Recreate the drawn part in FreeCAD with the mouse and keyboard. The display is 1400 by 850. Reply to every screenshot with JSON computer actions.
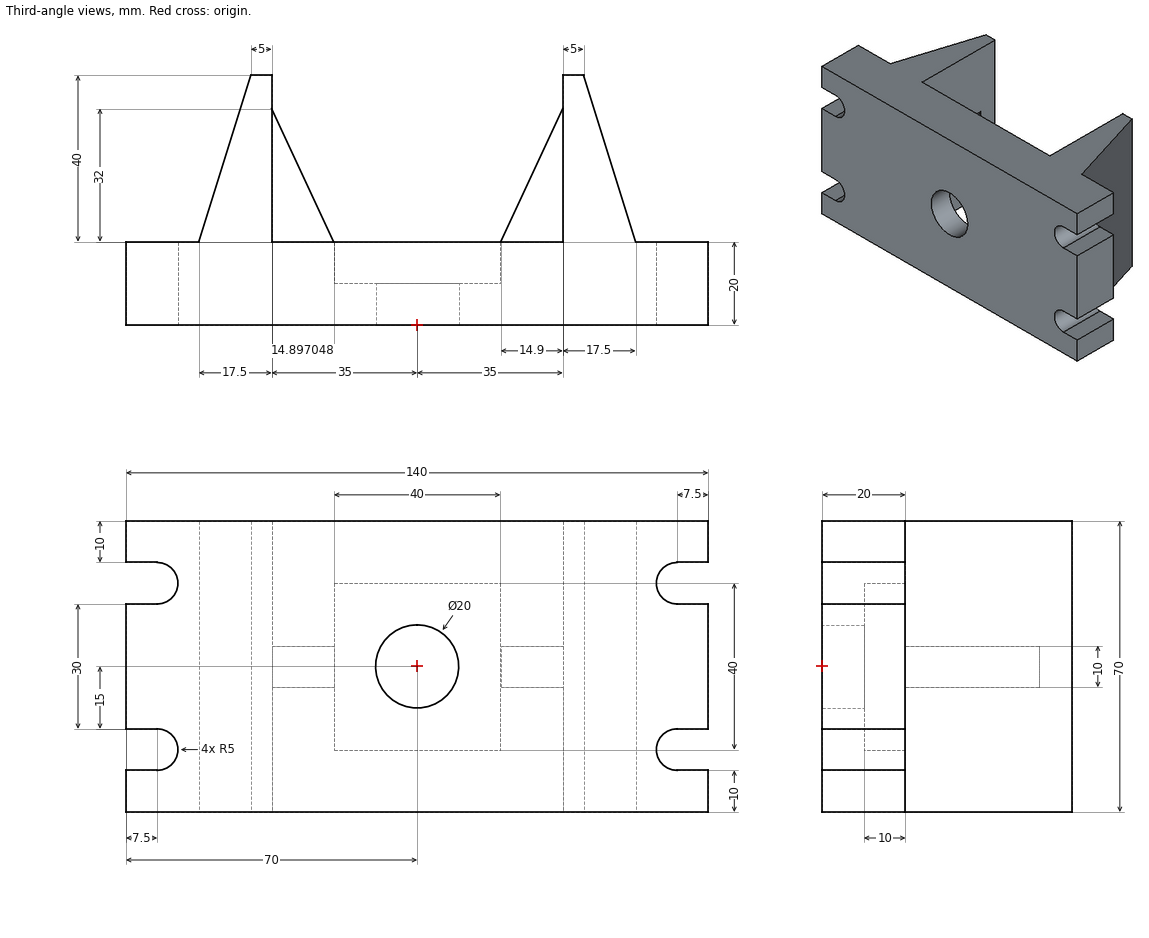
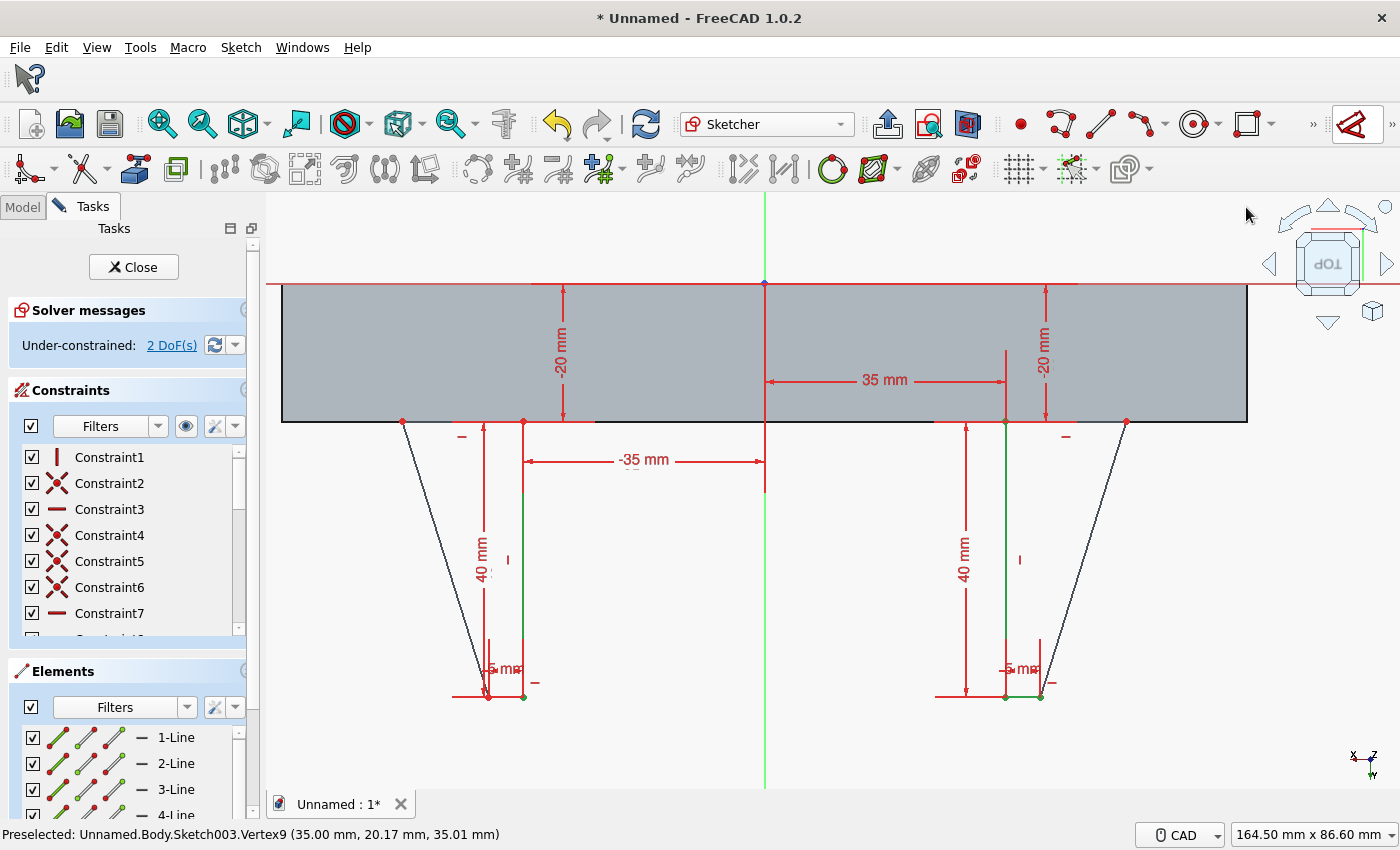
{"action": "left_click", "coordinate": [1090, 422]}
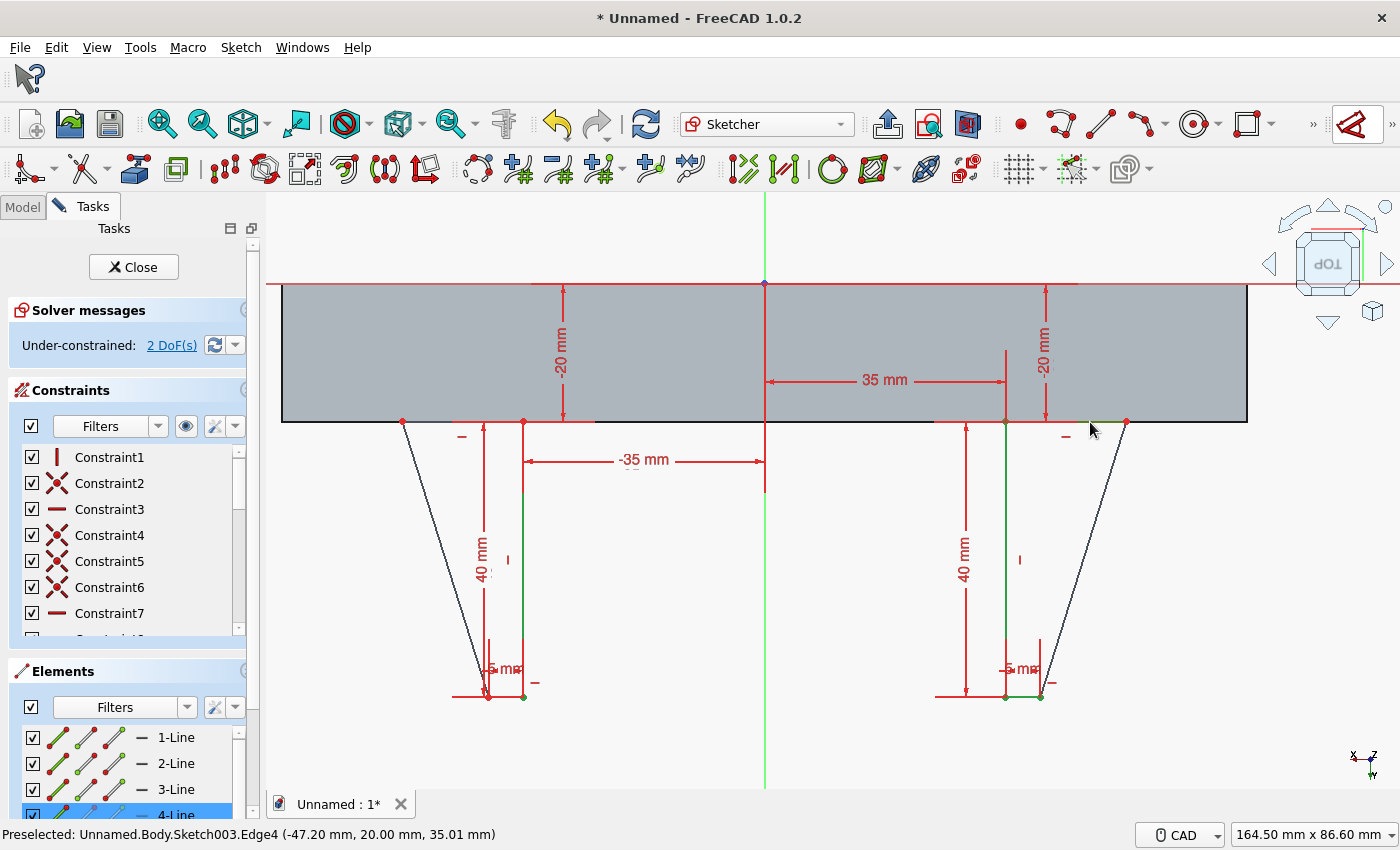
{"action": "left_click", "coordinate": [1378, 124]}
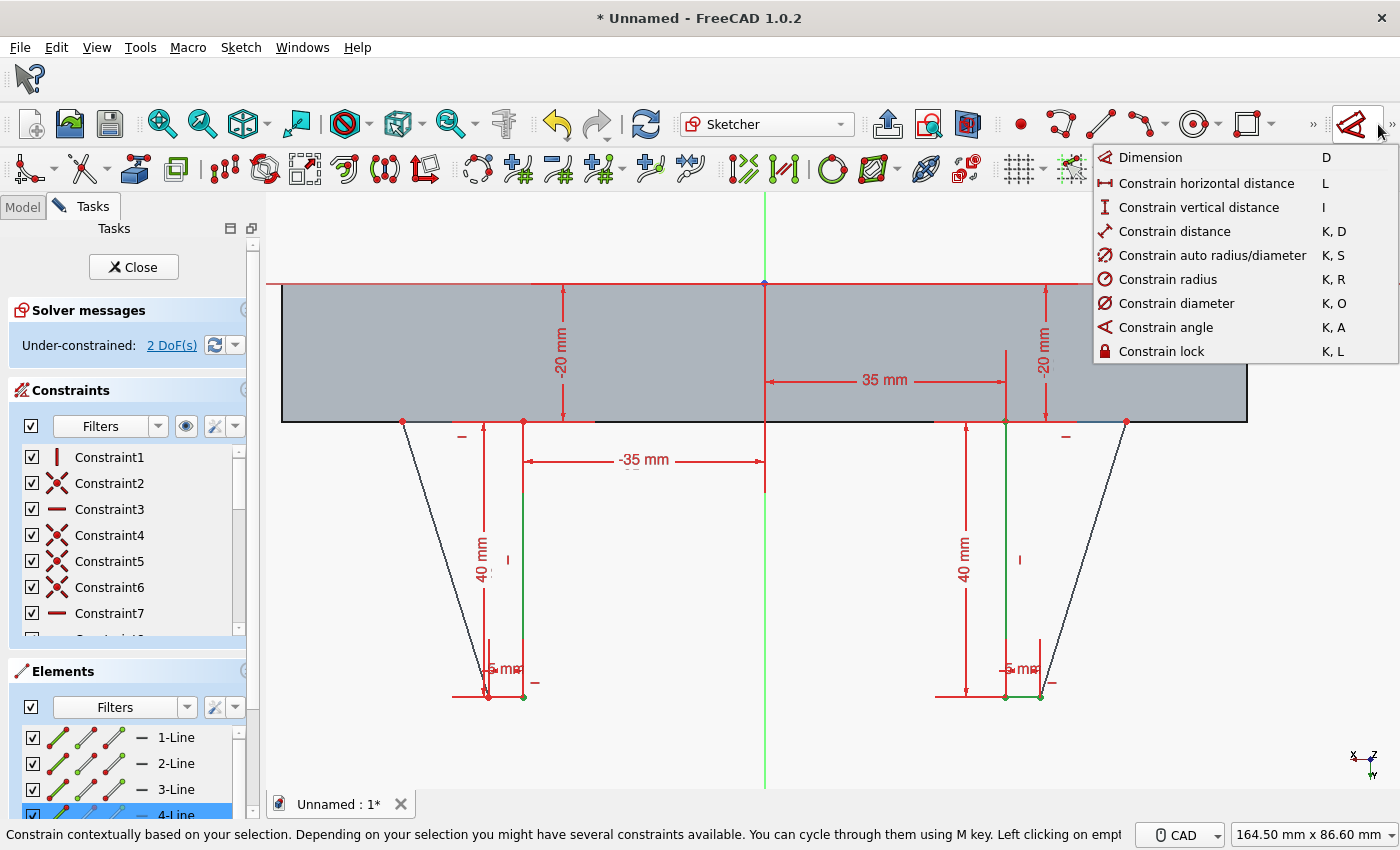
{"action": "left_click", "coordinate": [1246, 183]}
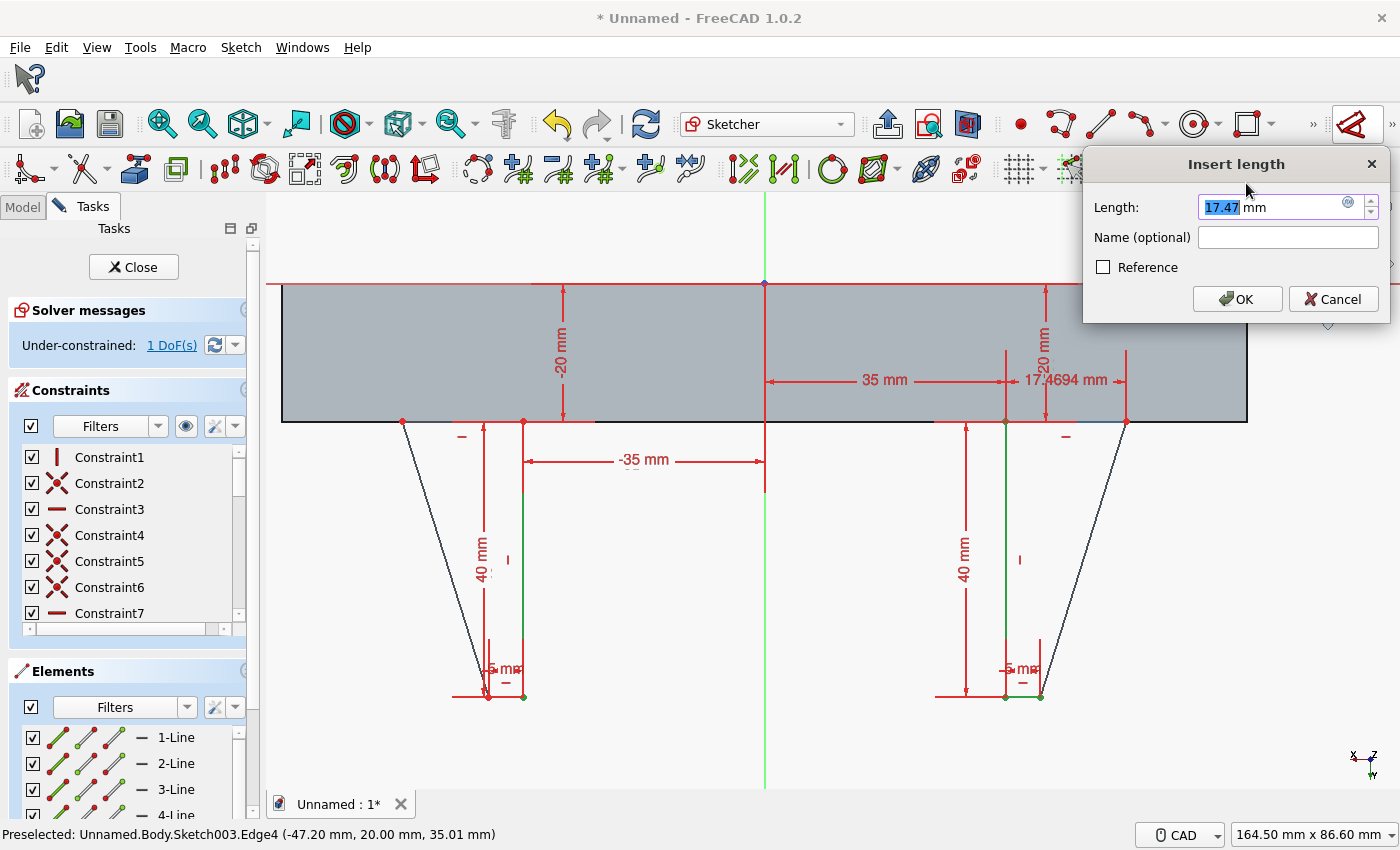
{"action": "type", "text": "17.5"}
{"action": "key", "text": "Return"}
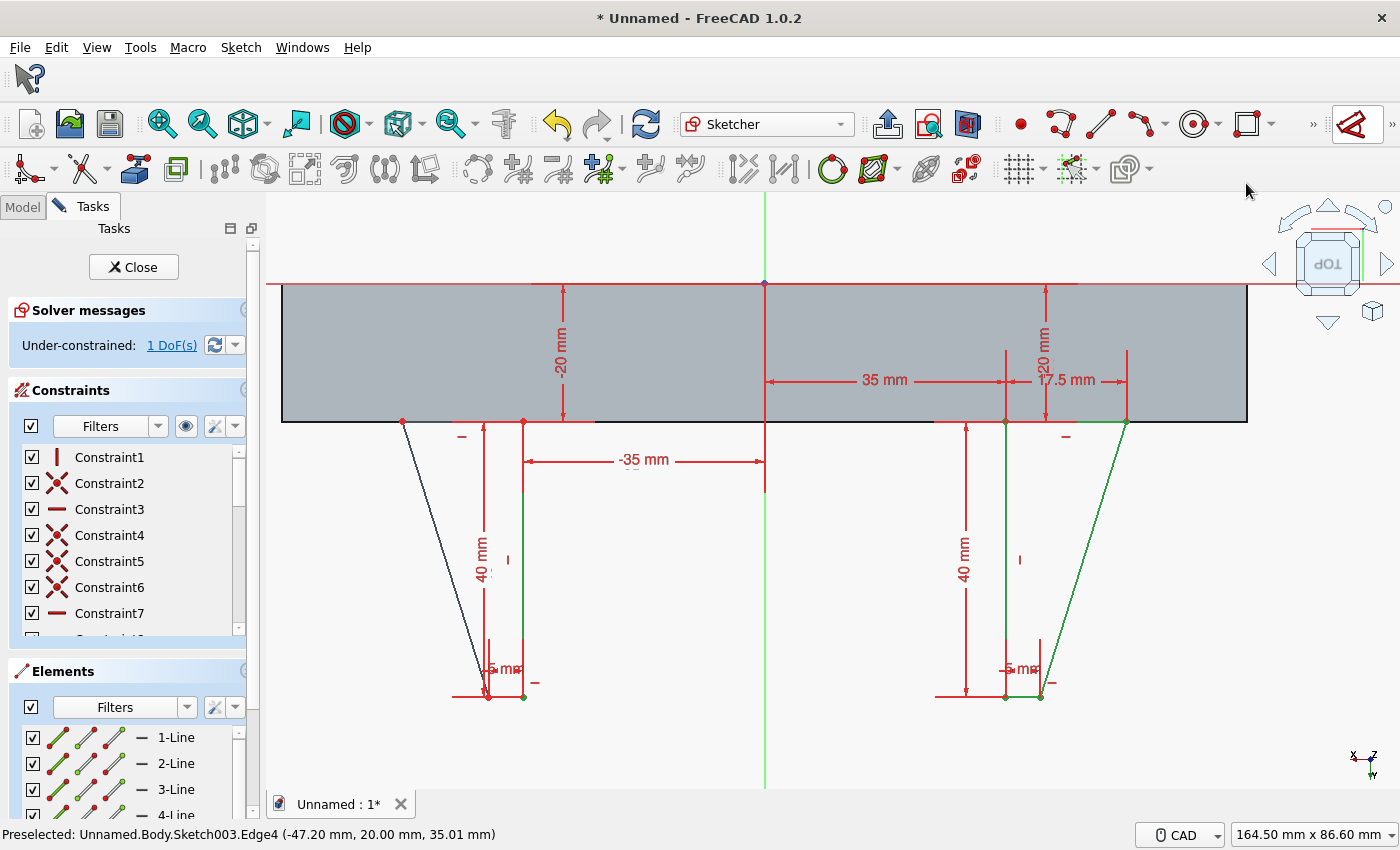
{"action": "left_click", "coordinate": [487, 422]}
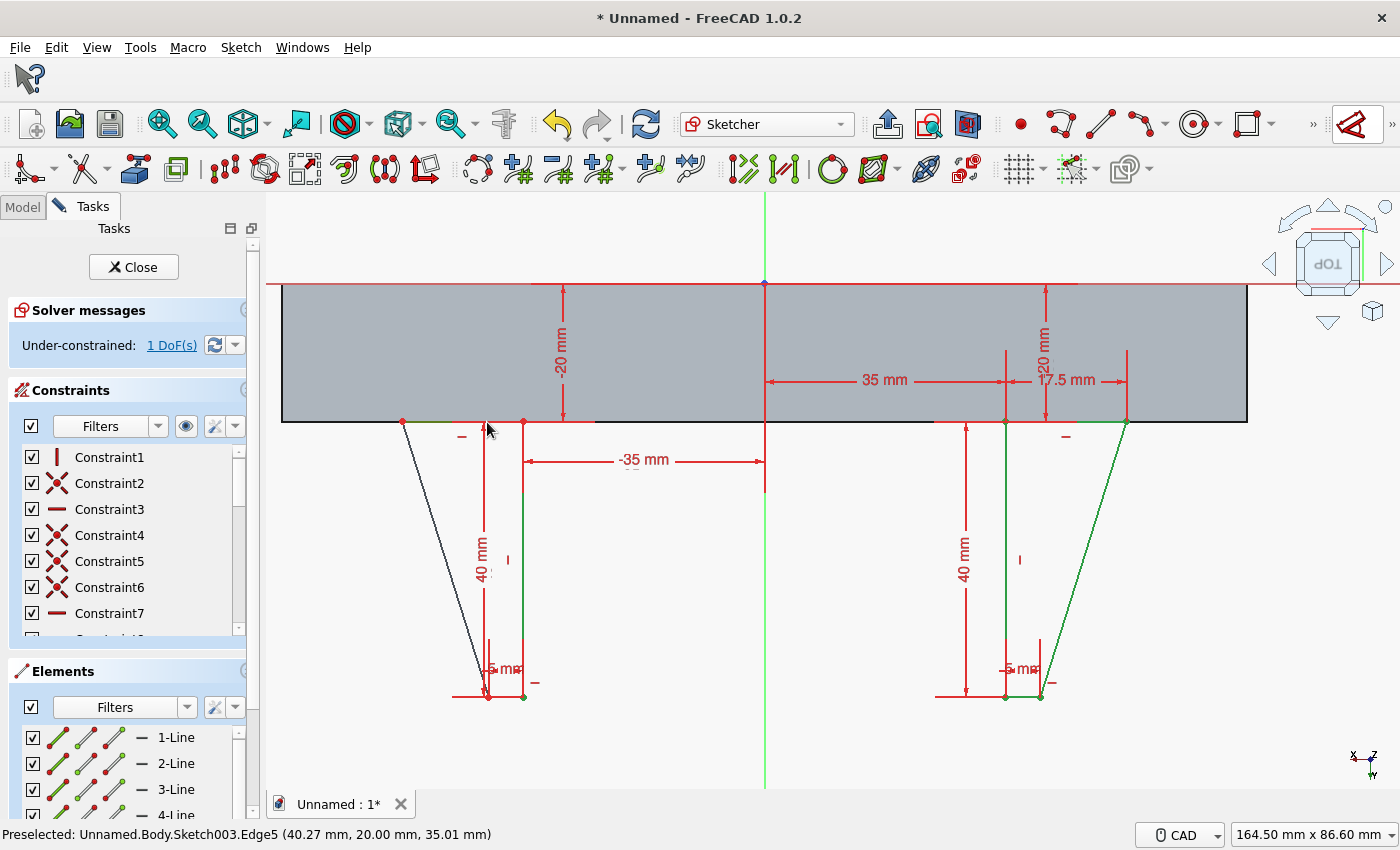
{"action": "key", "text": "l"}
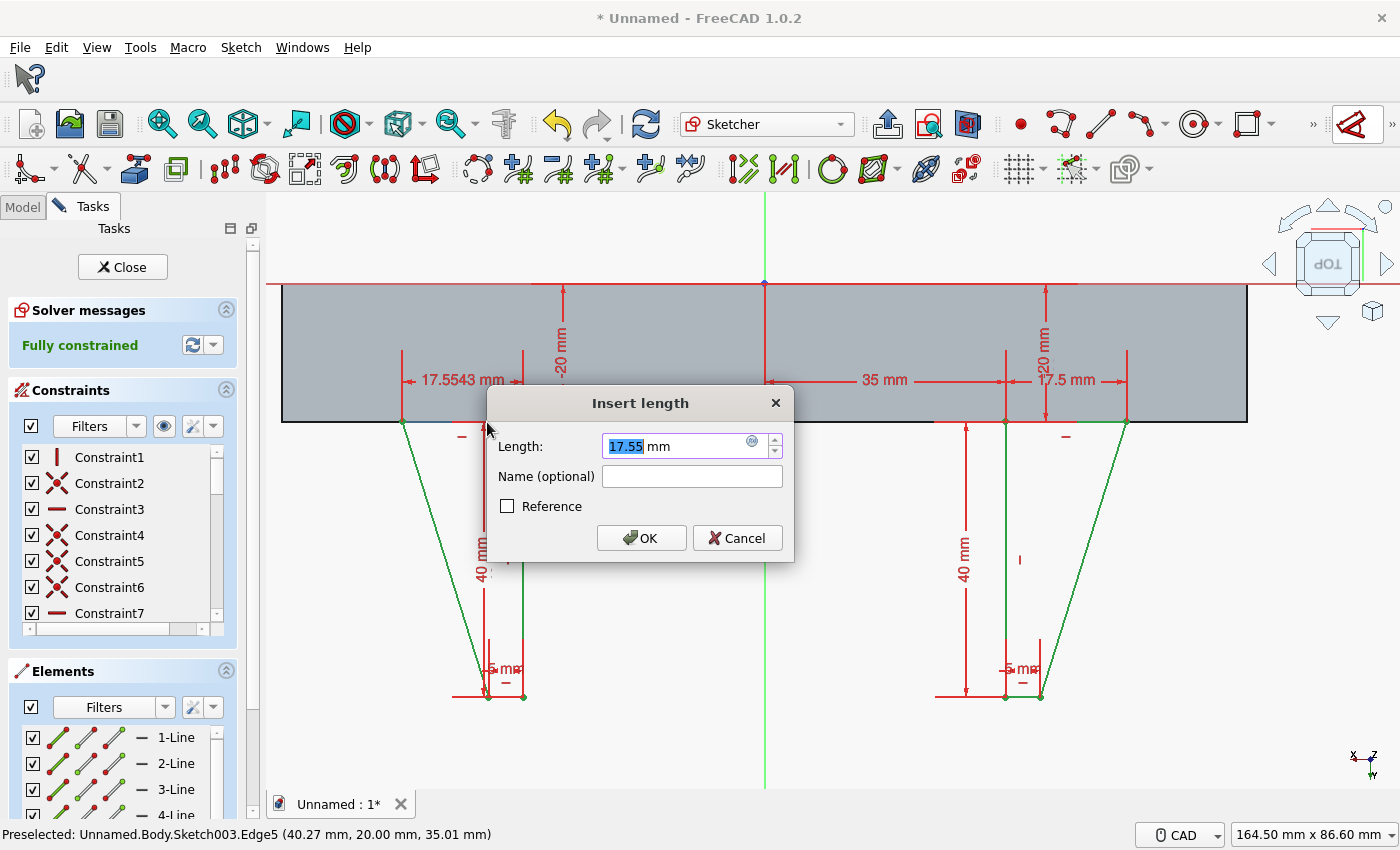
{"action": "type", "text": "17.5"}
{"action": "key", "text": "Return"}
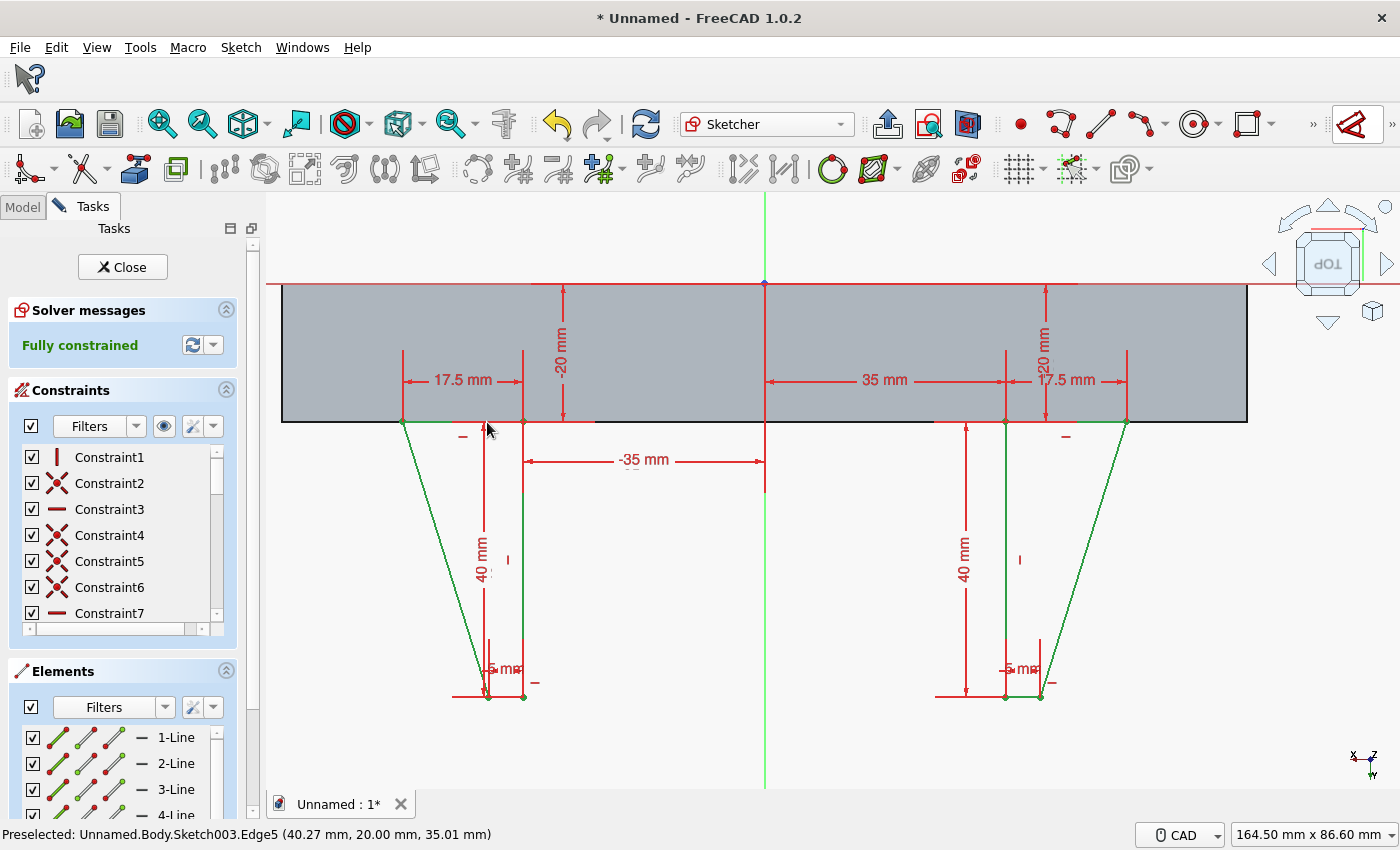
{"action": "left_click", "coordinate": [123, 267]}